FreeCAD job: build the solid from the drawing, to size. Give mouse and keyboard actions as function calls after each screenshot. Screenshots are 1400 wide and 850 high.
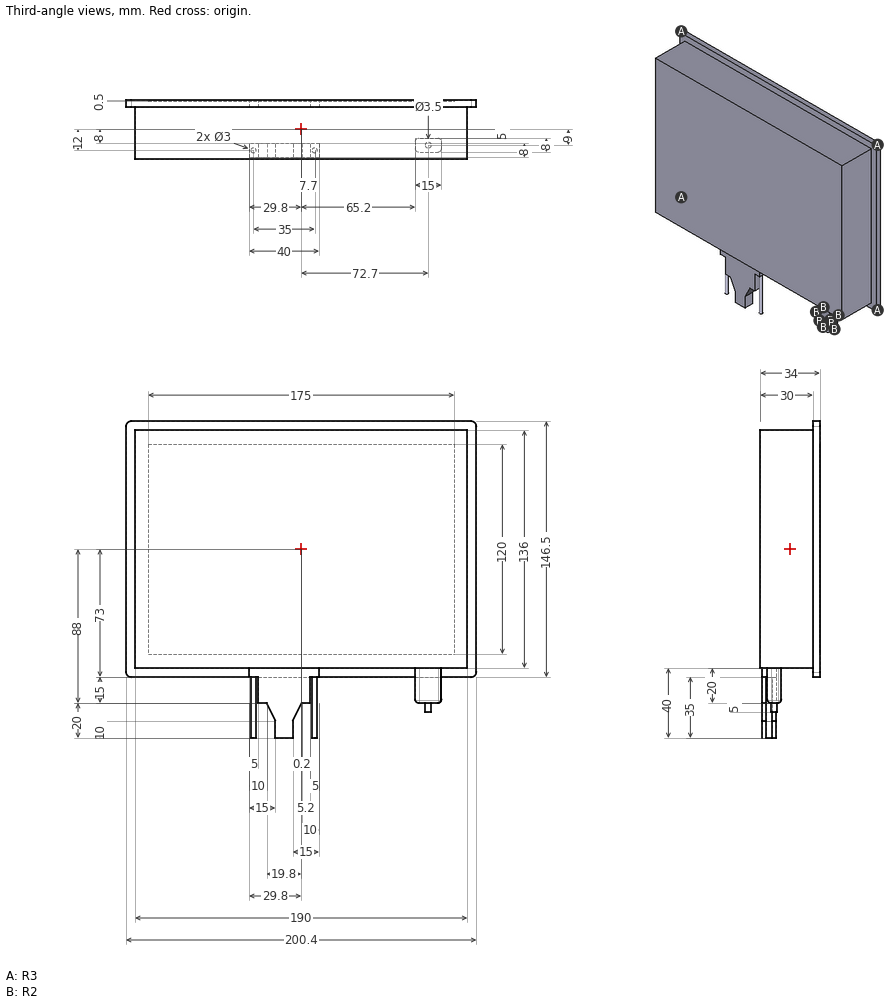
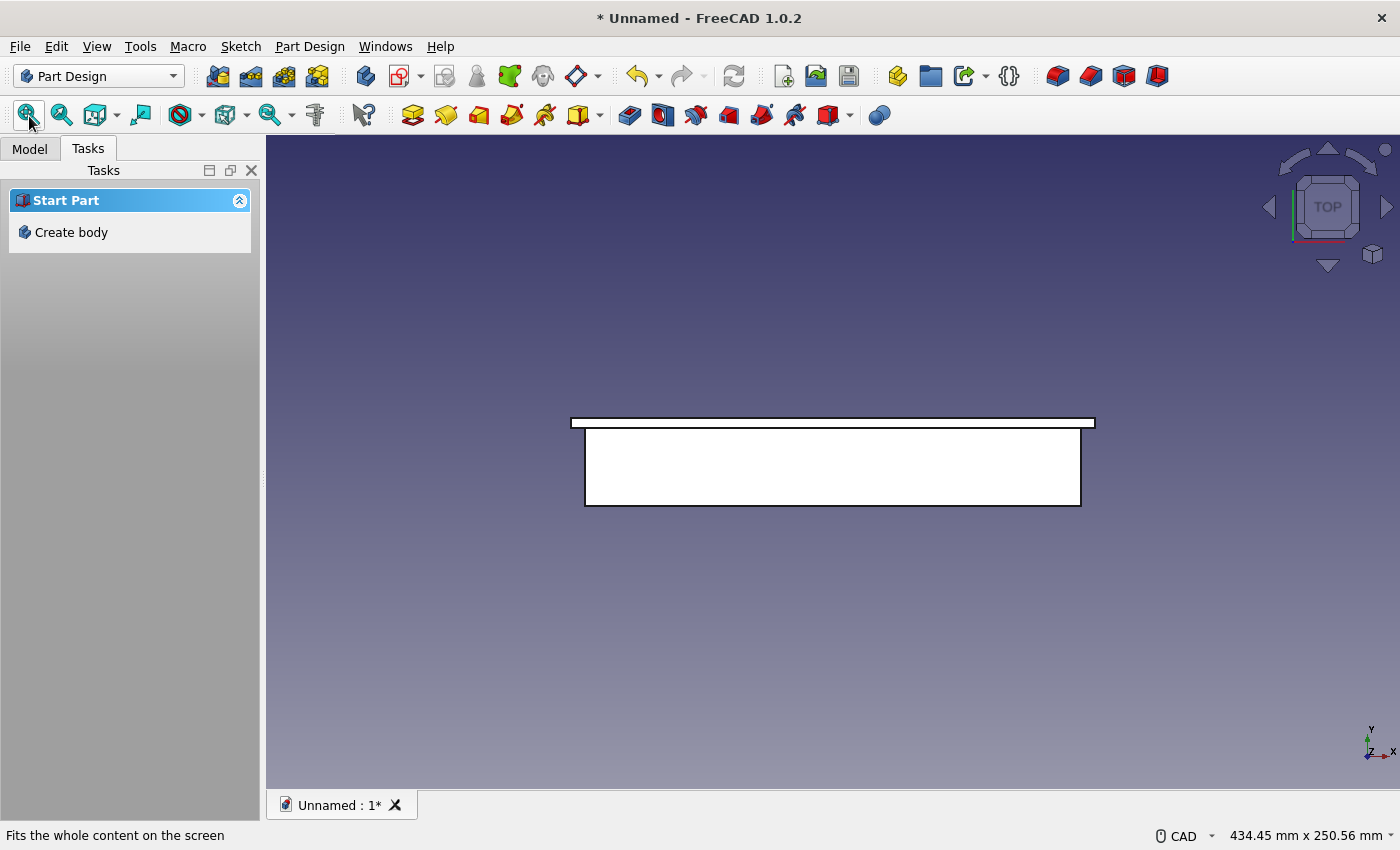
click(1095, 423)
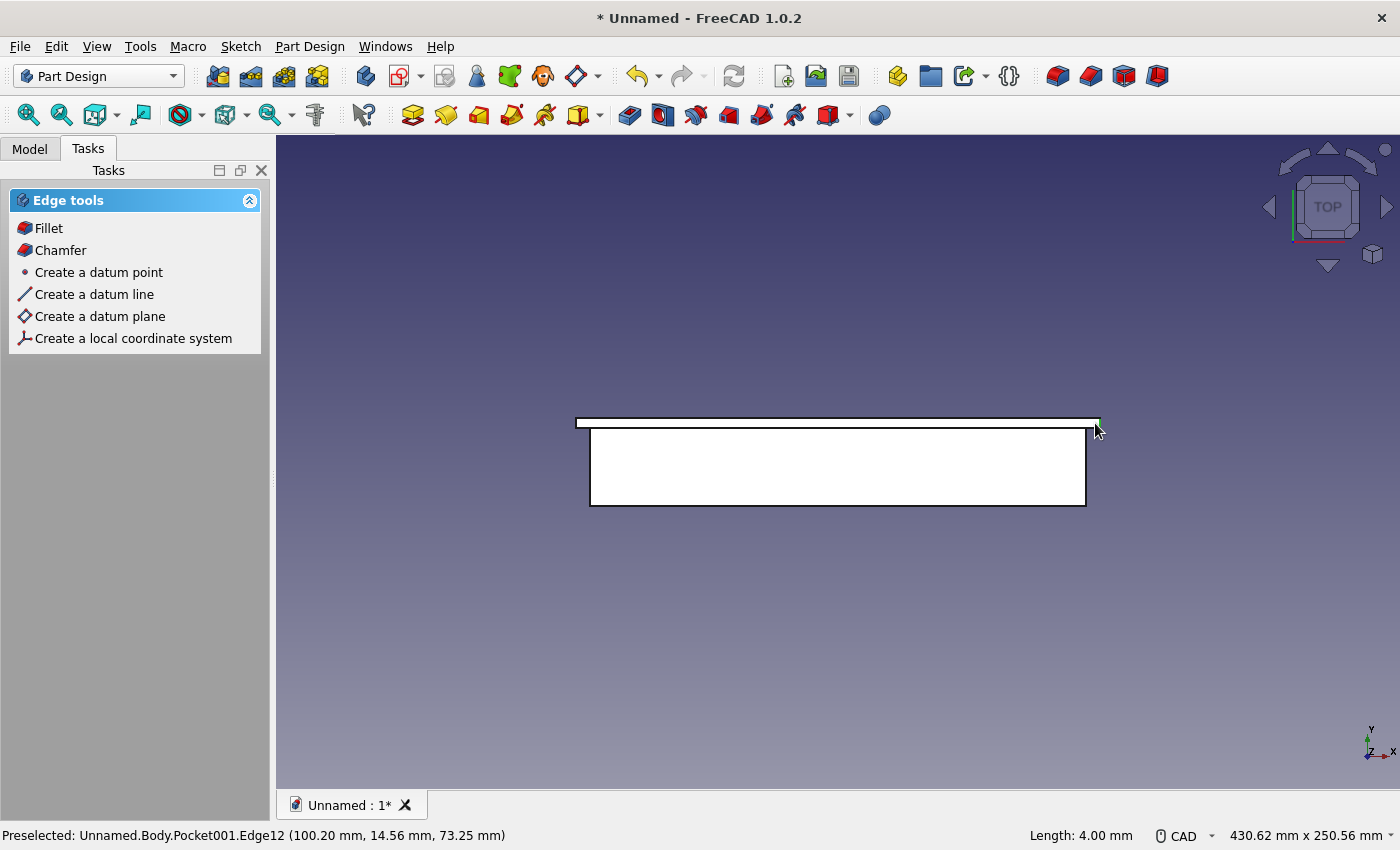
click(576, 423, ctrl)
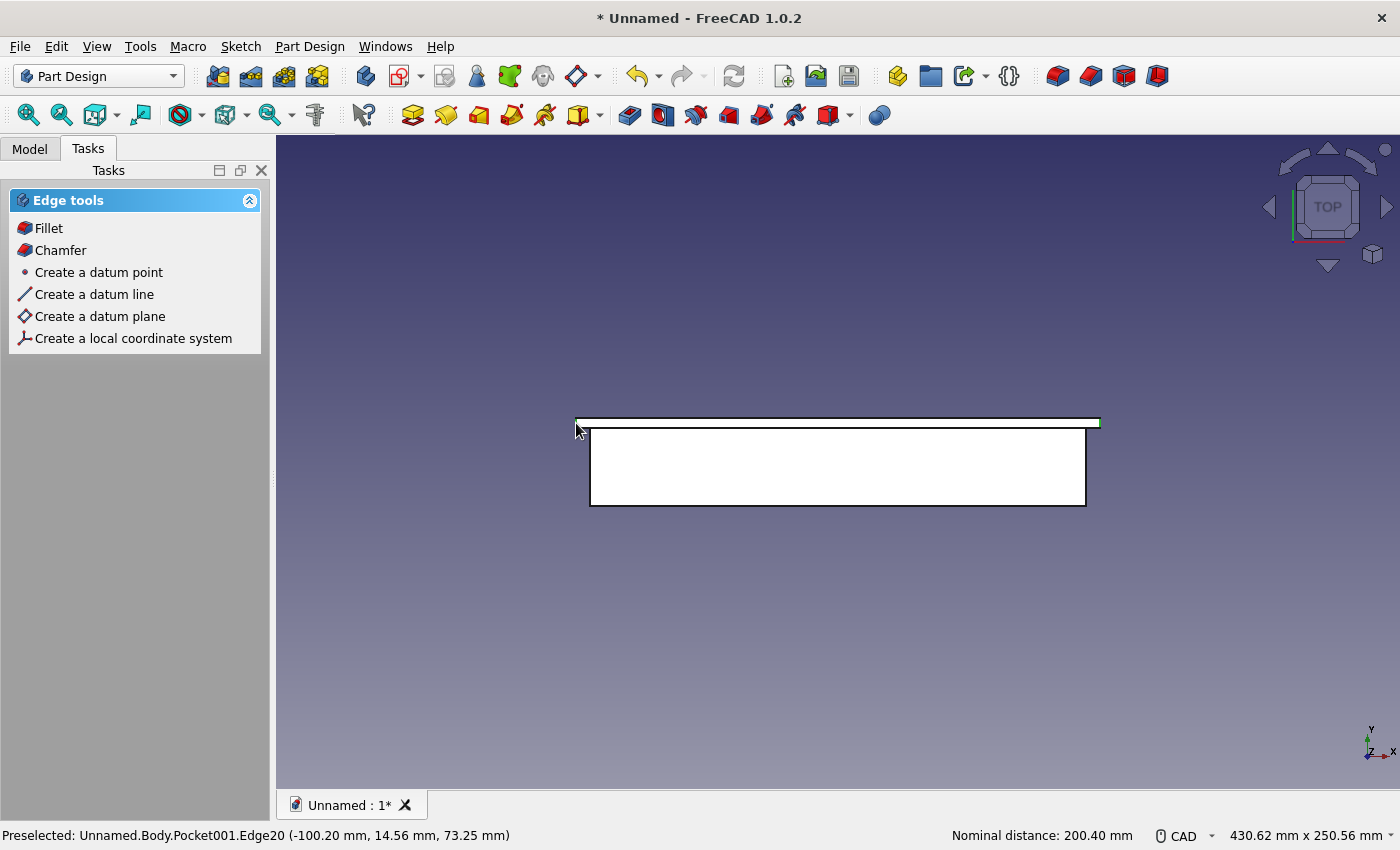
scroll(576, 422, up, 7)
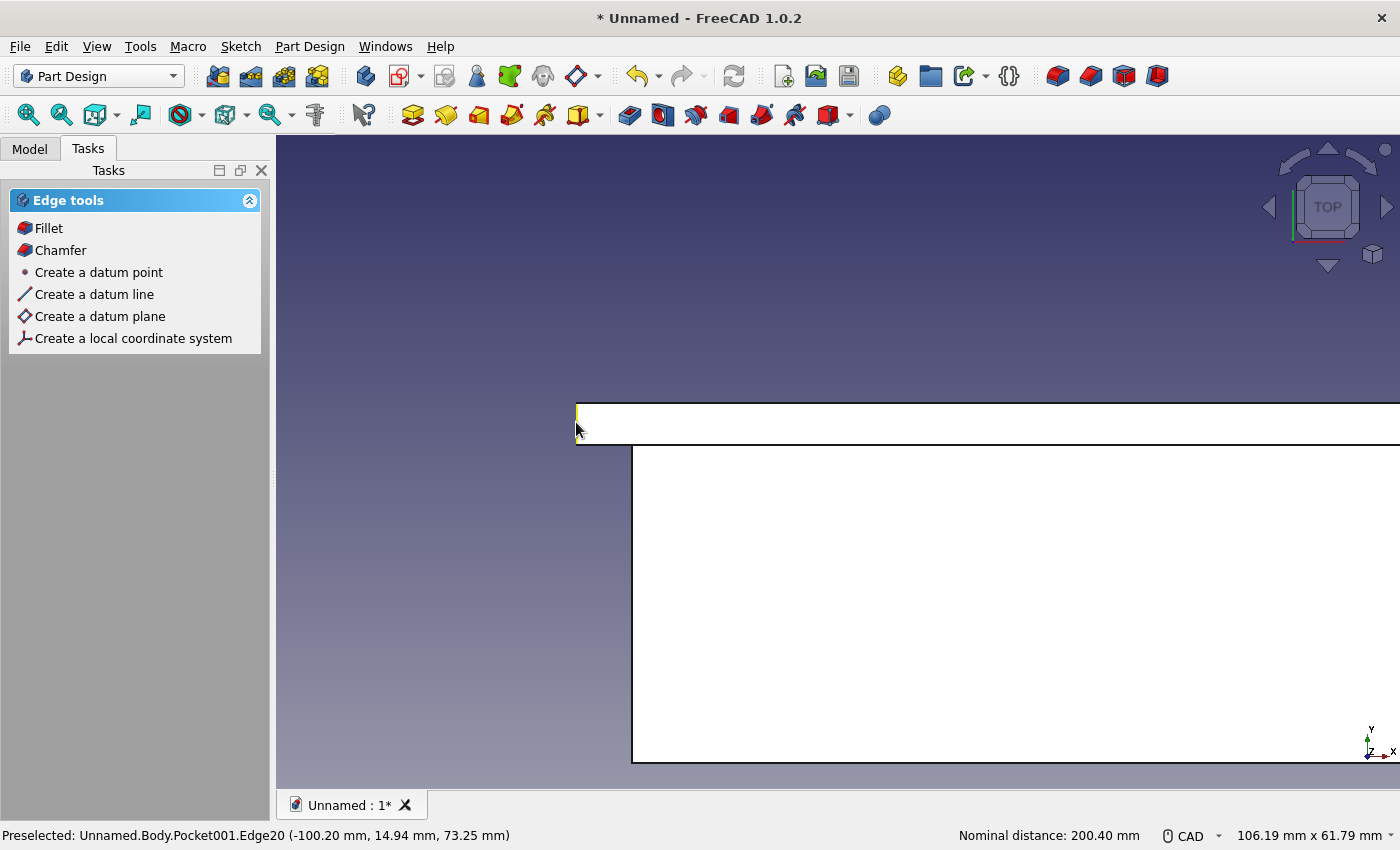
click(29, 116)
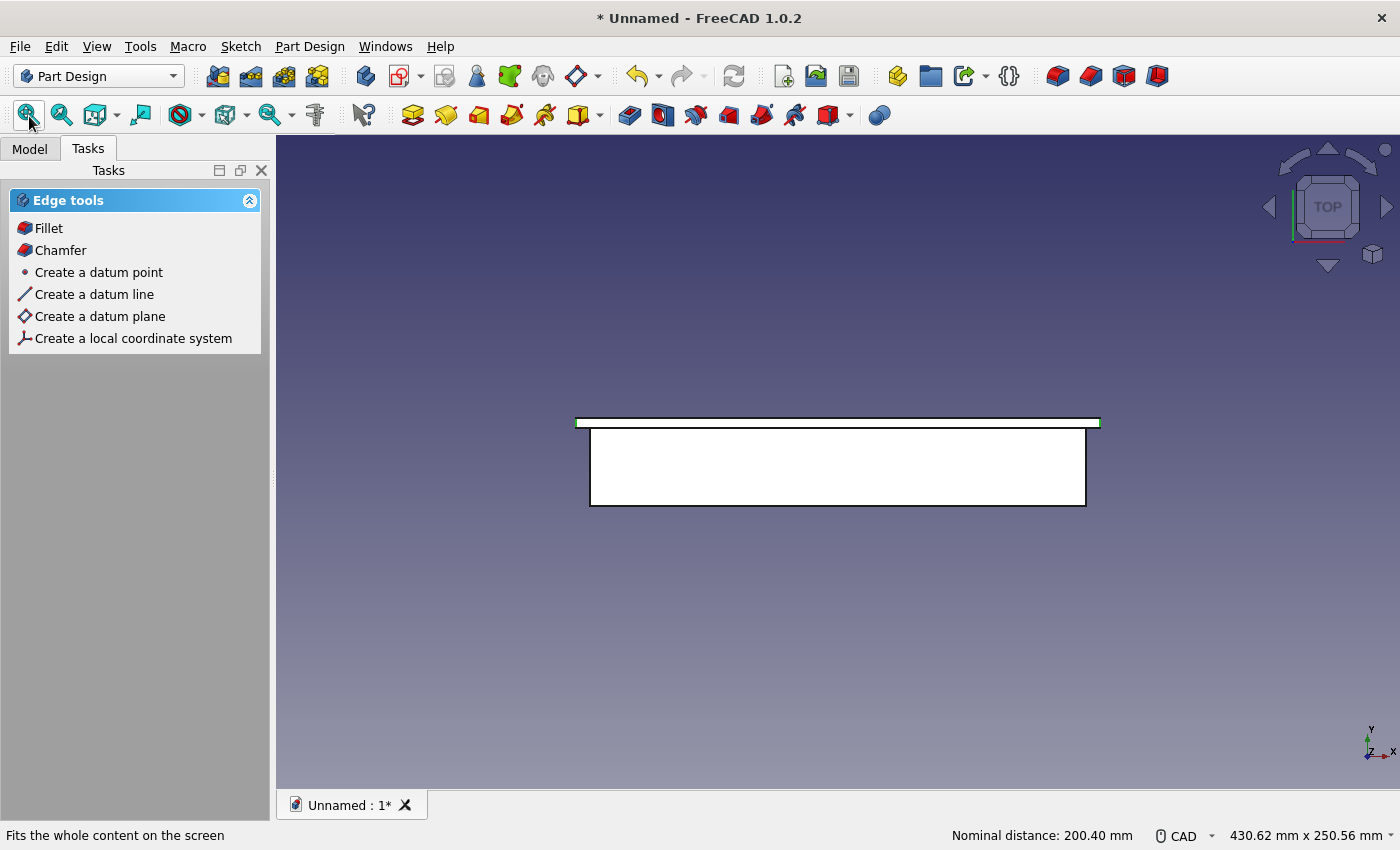
key(0)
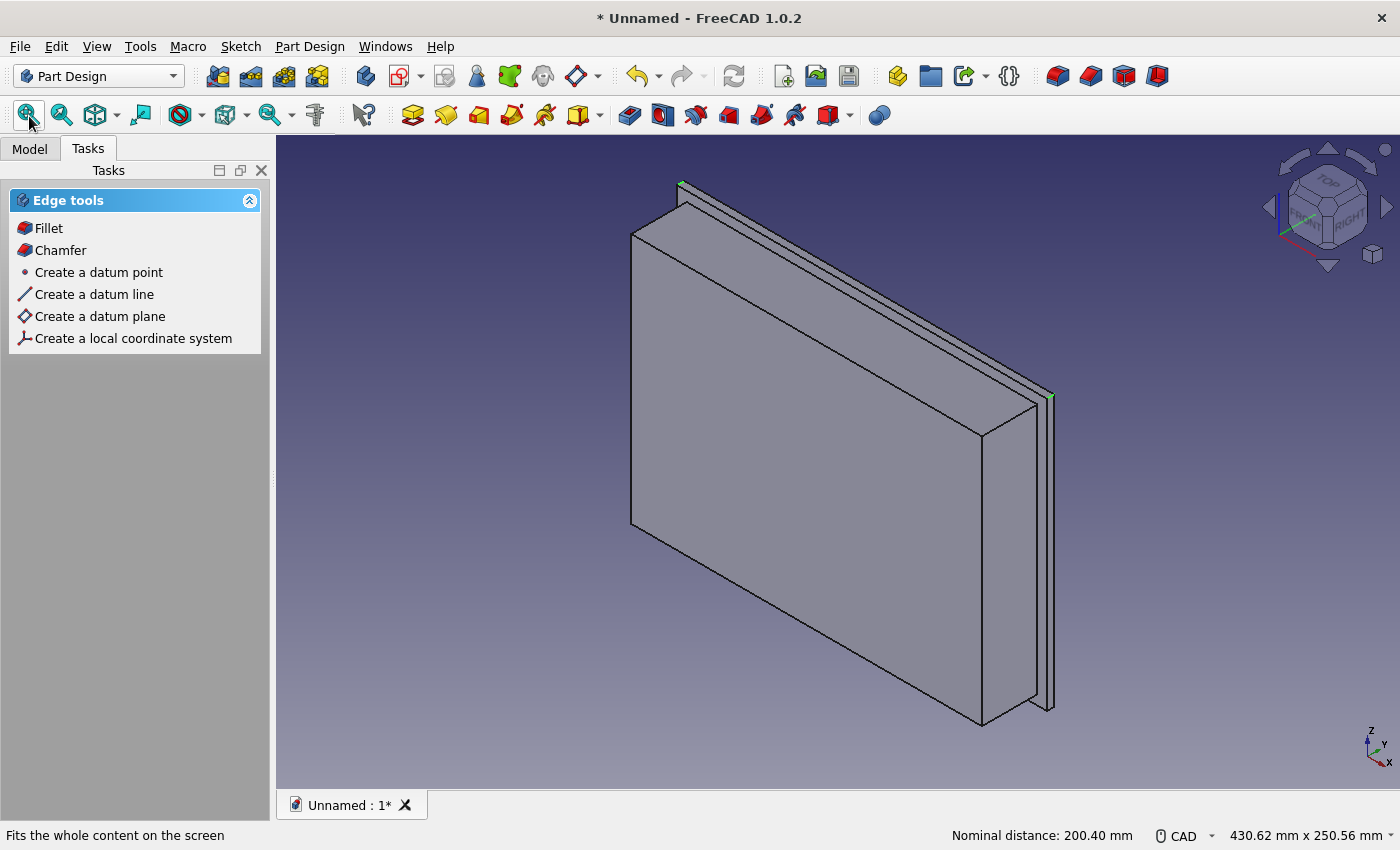
scroll(681, 494, up, 7)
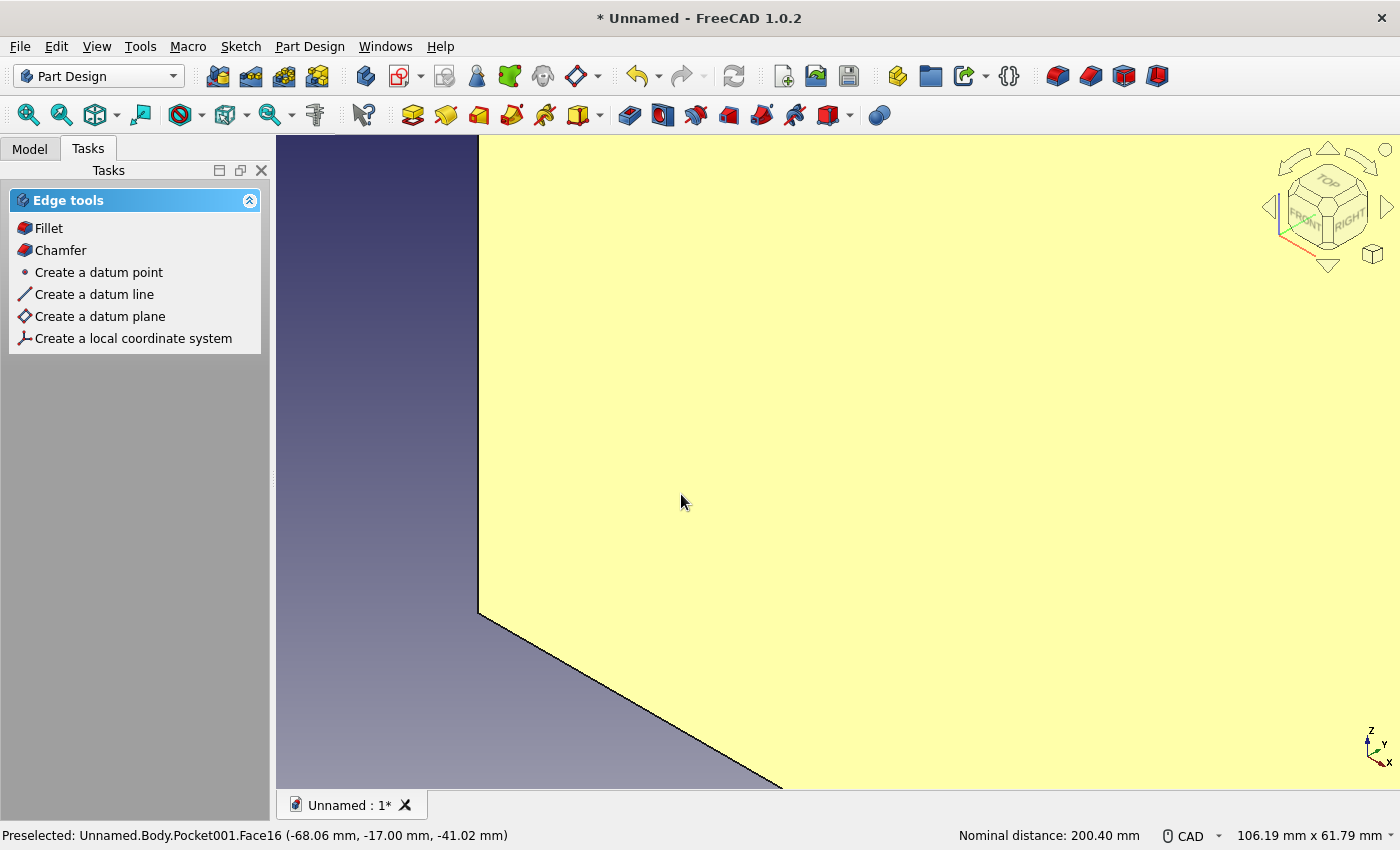
click(29, 116)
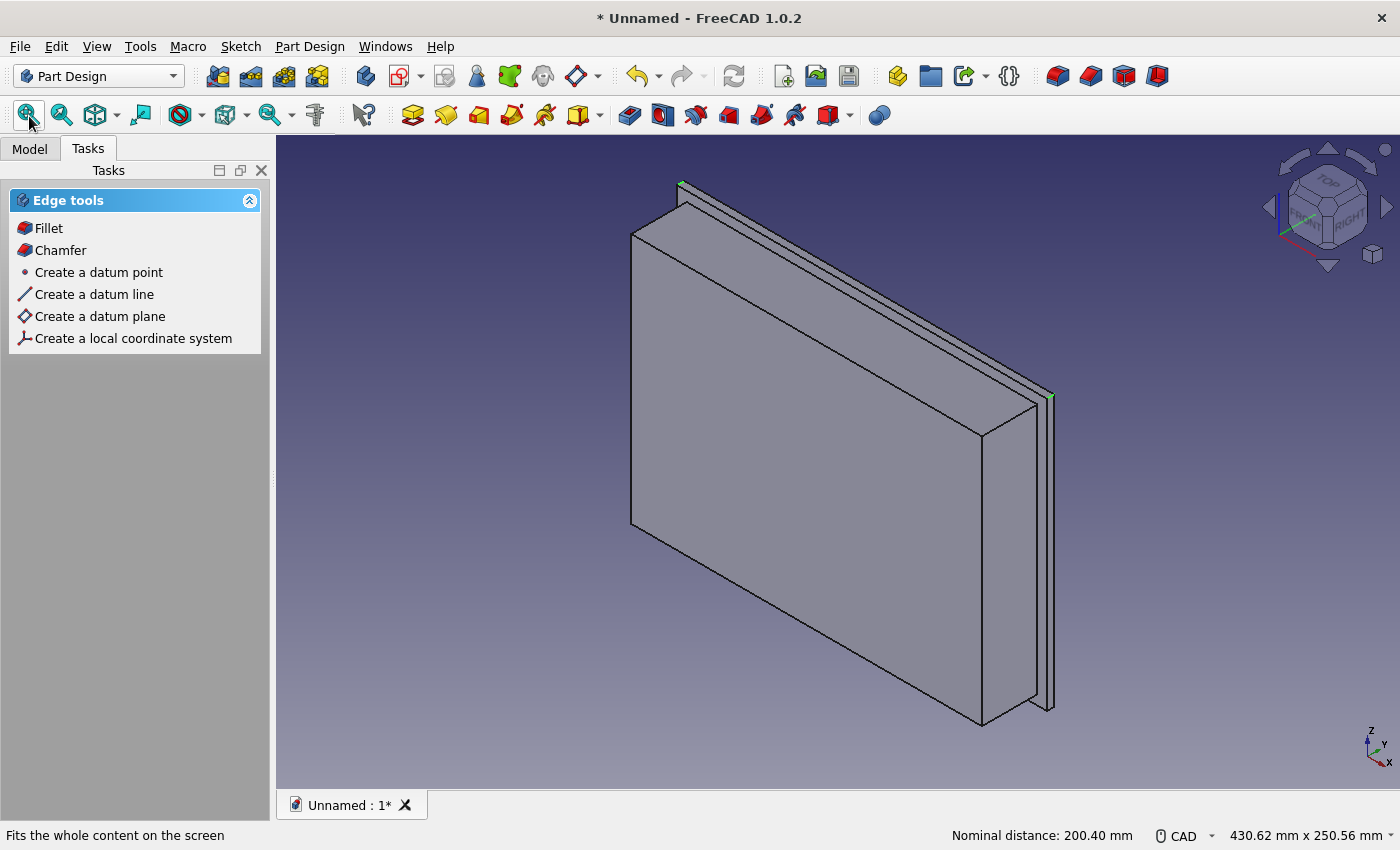
key(1)